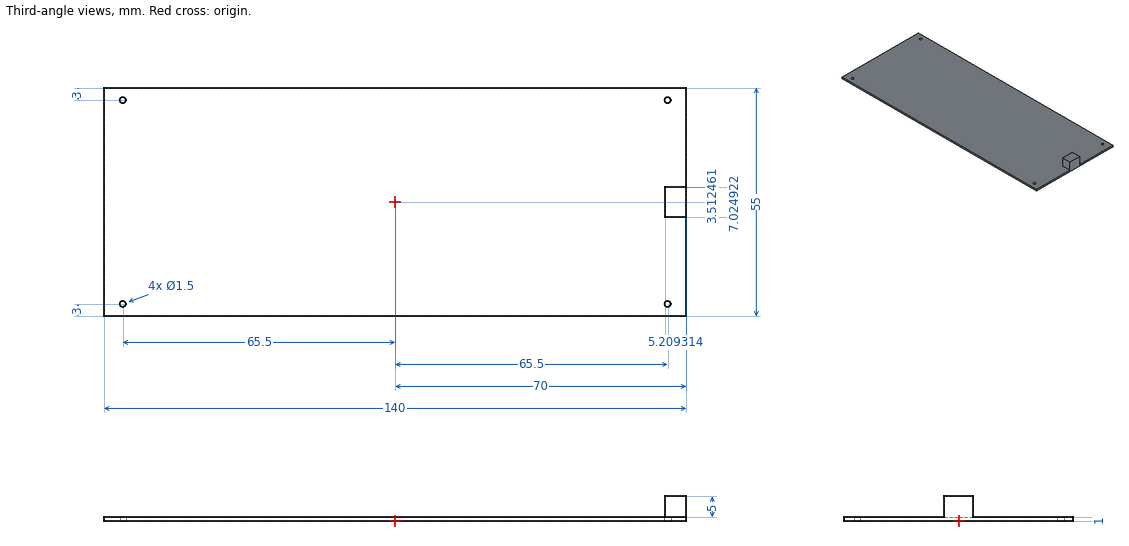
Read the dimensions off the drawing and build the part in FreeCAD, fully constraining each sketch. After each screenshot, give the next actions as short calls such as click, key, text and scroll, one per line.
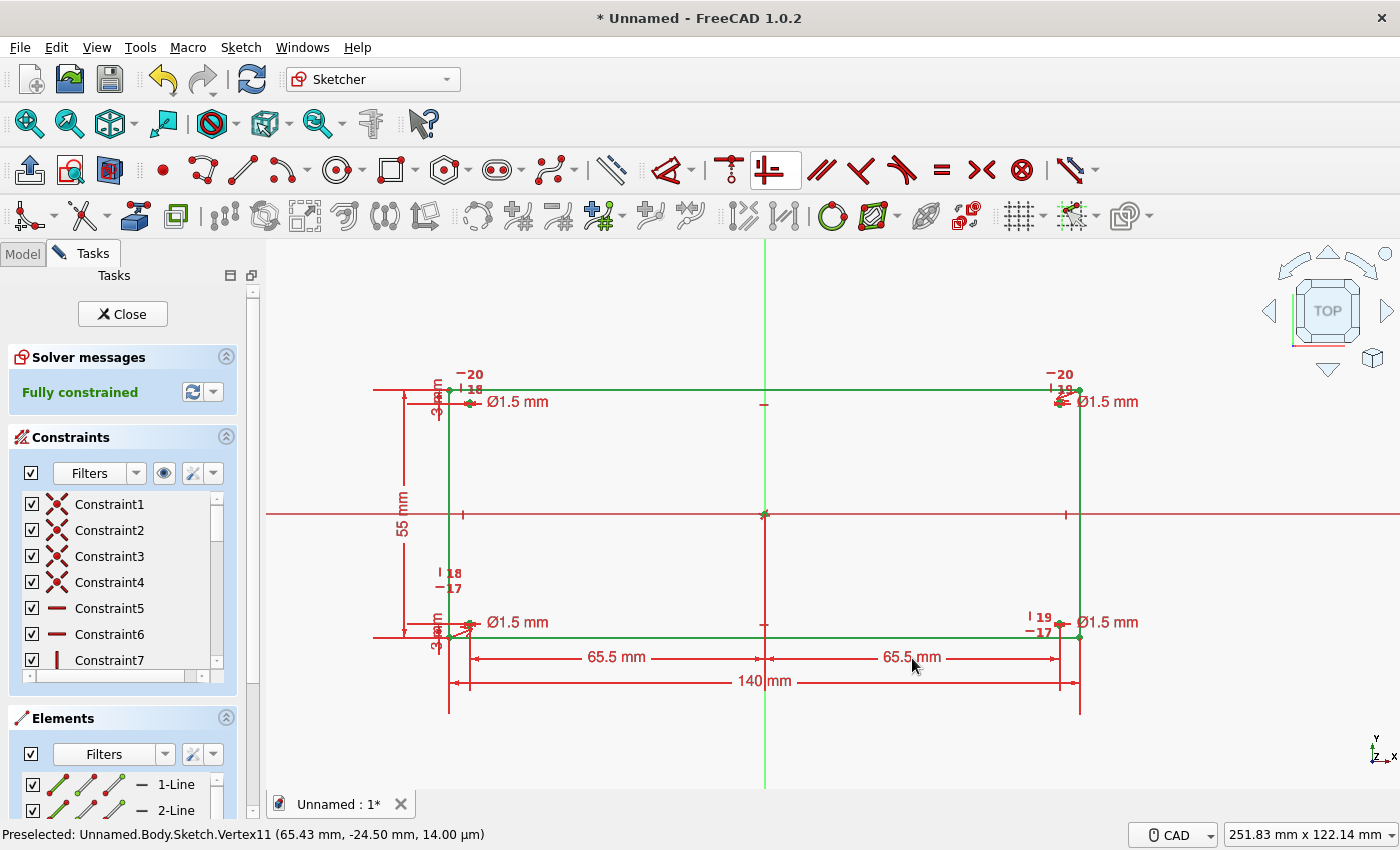
click(123, 314)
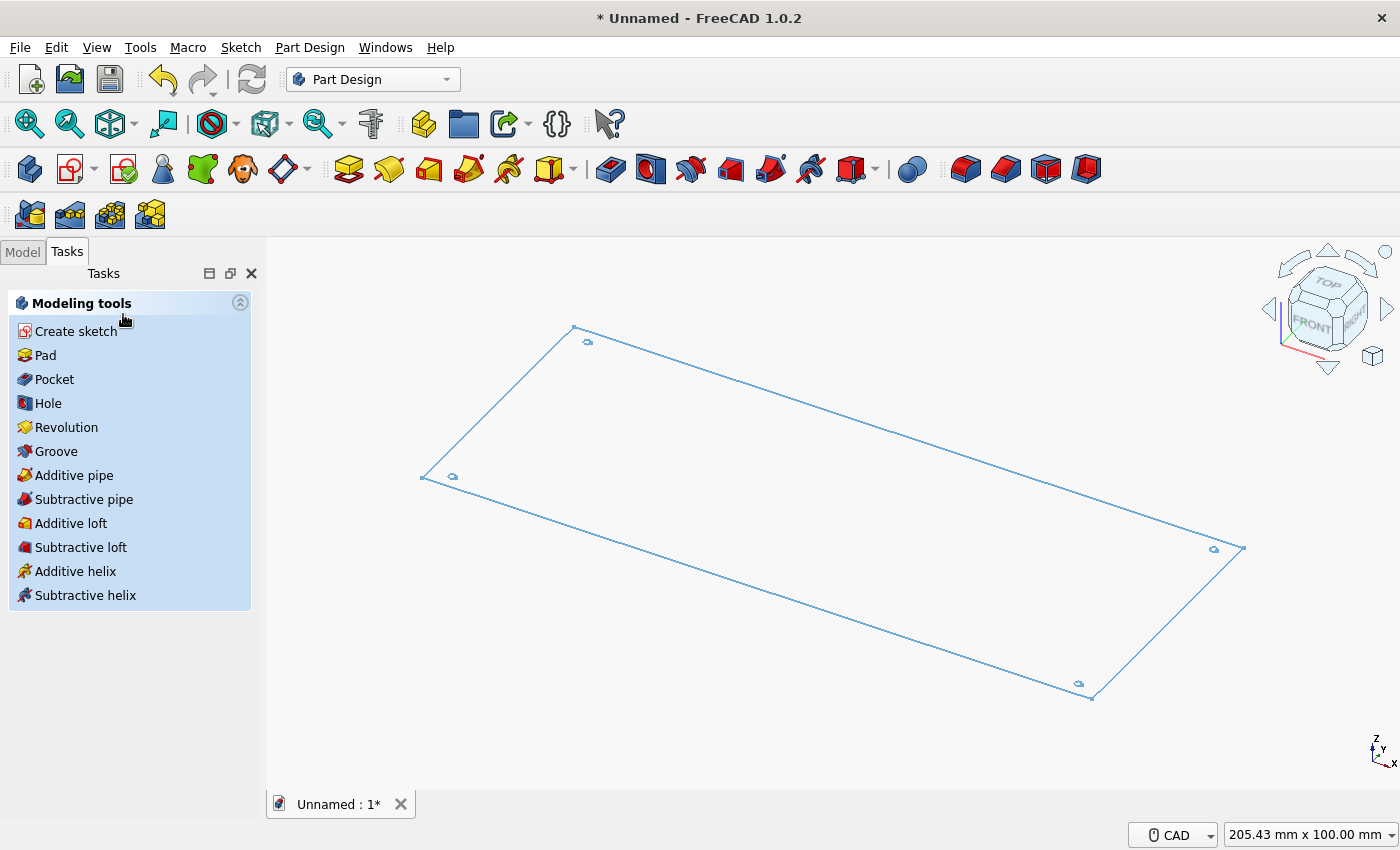
click(350, 170)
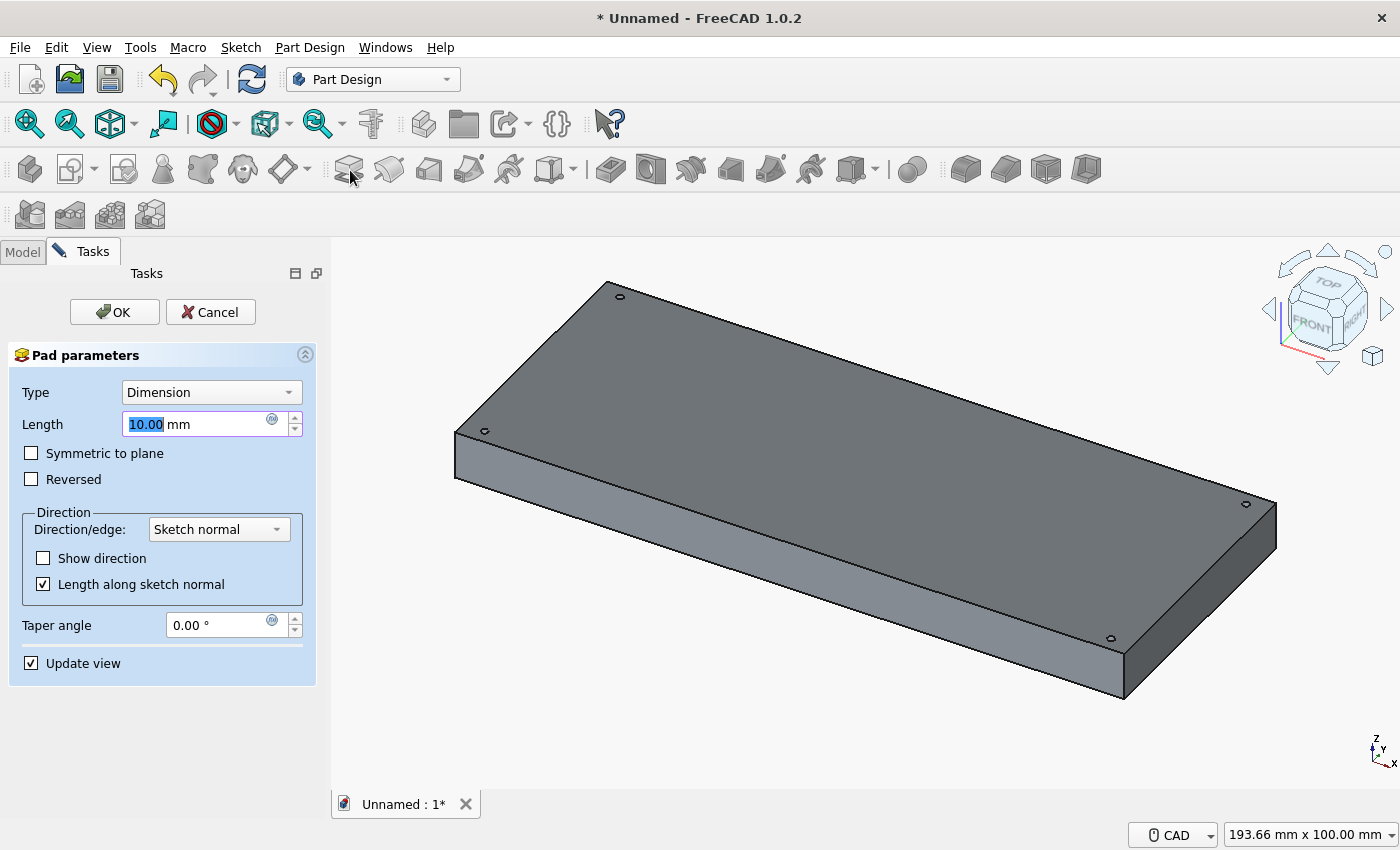
text(1)
key(Tab)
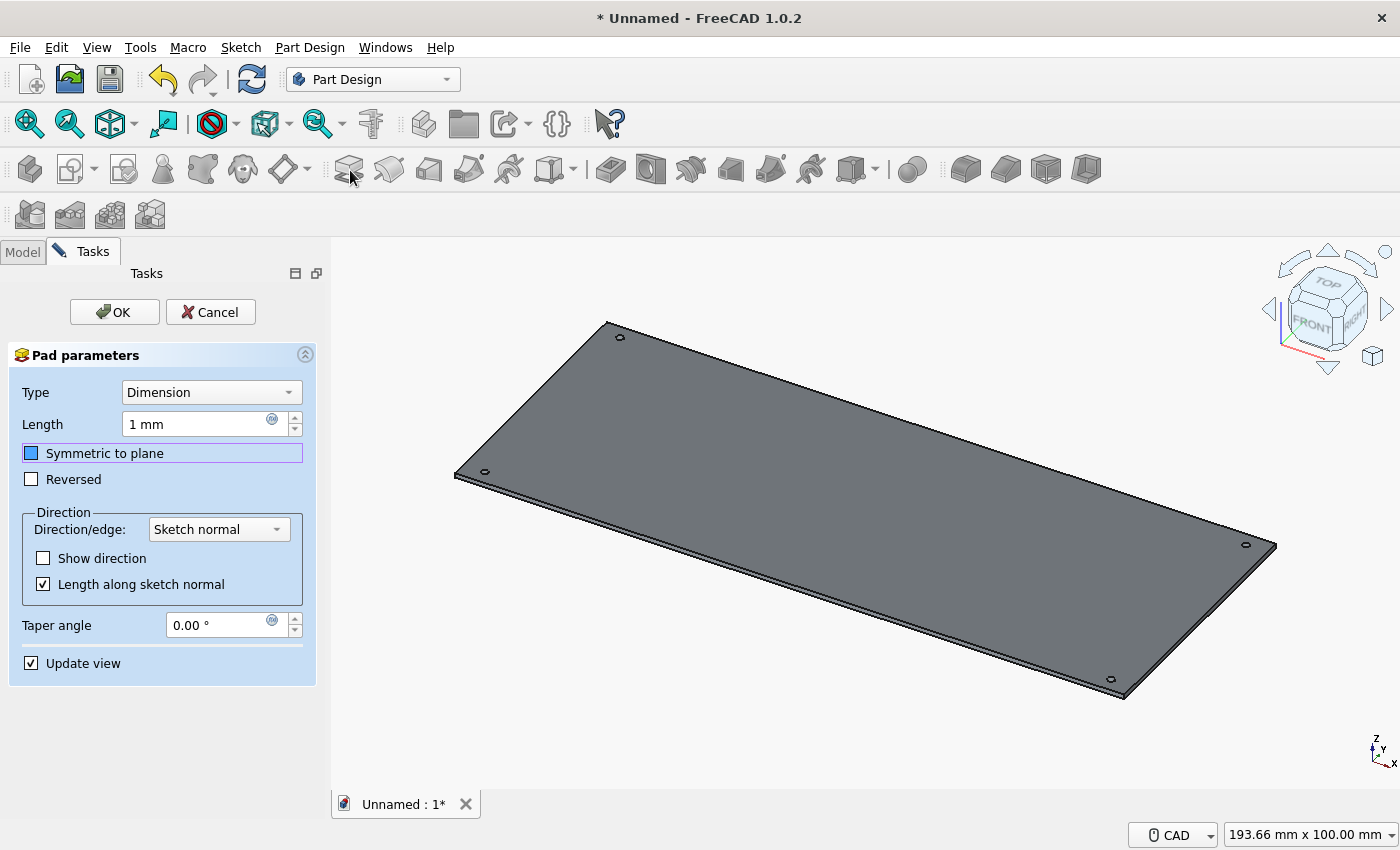
click(115, 312)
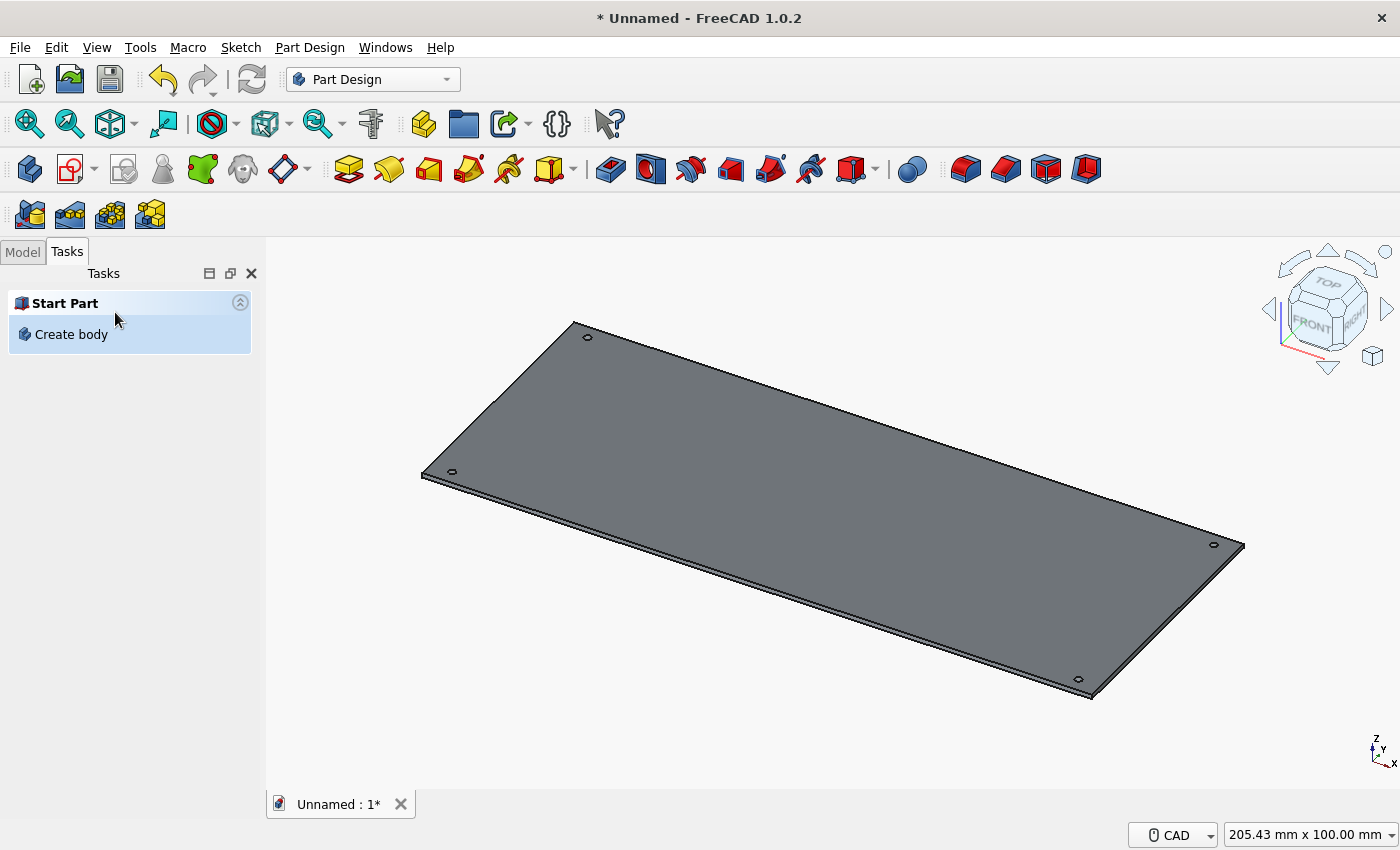
click(1024, 571)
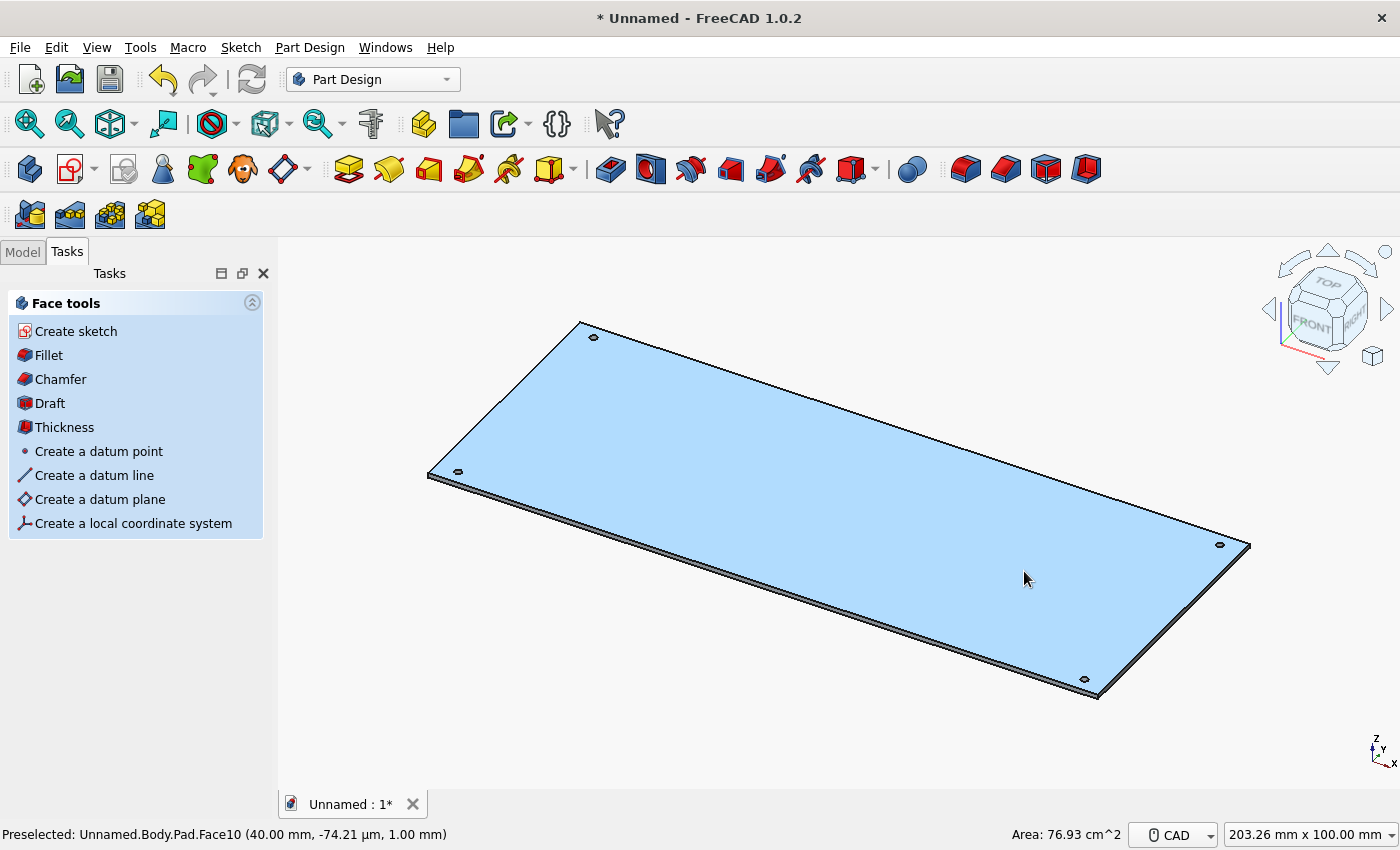
click(70, 170)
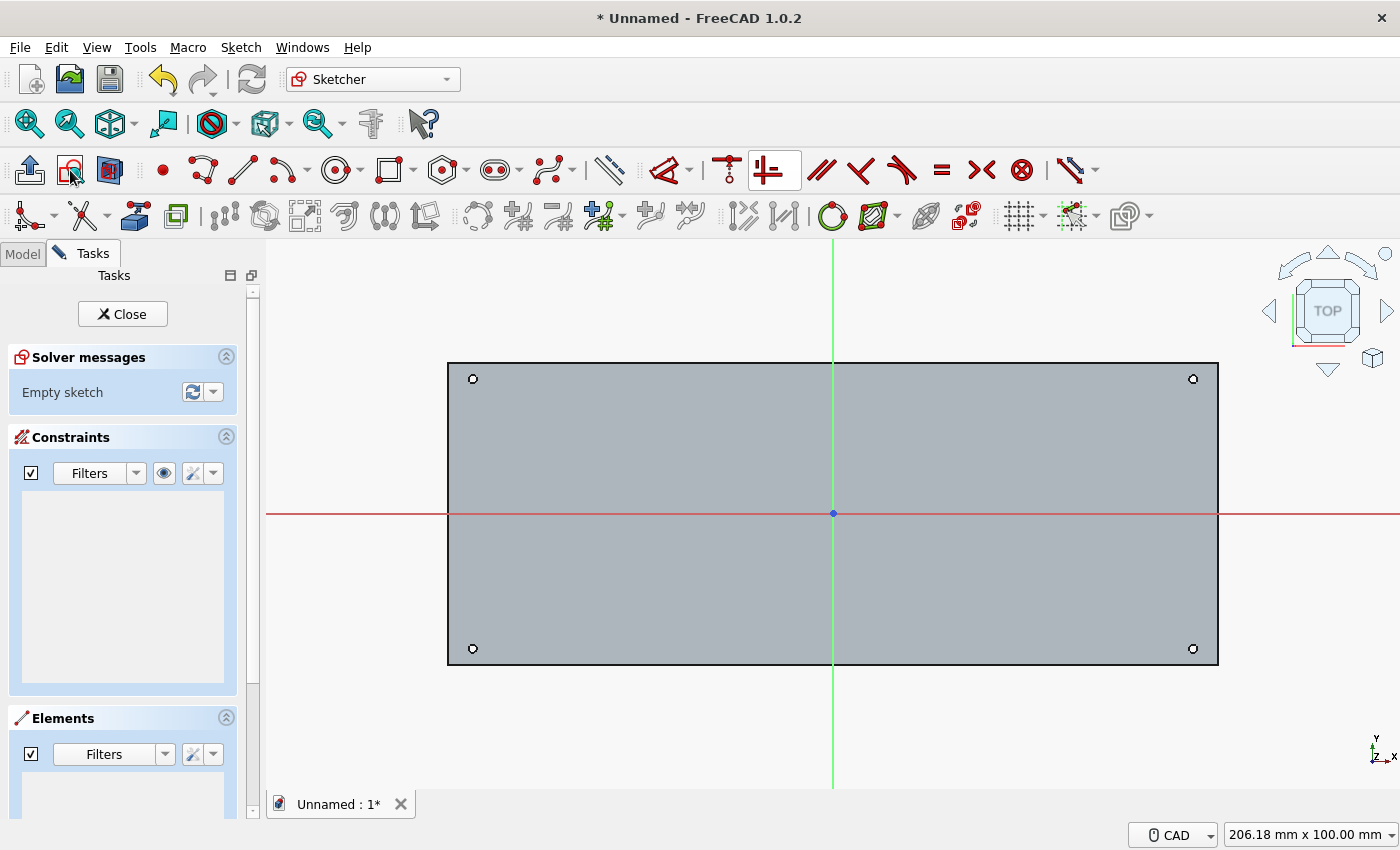
scroll(1235, 514, up, 11)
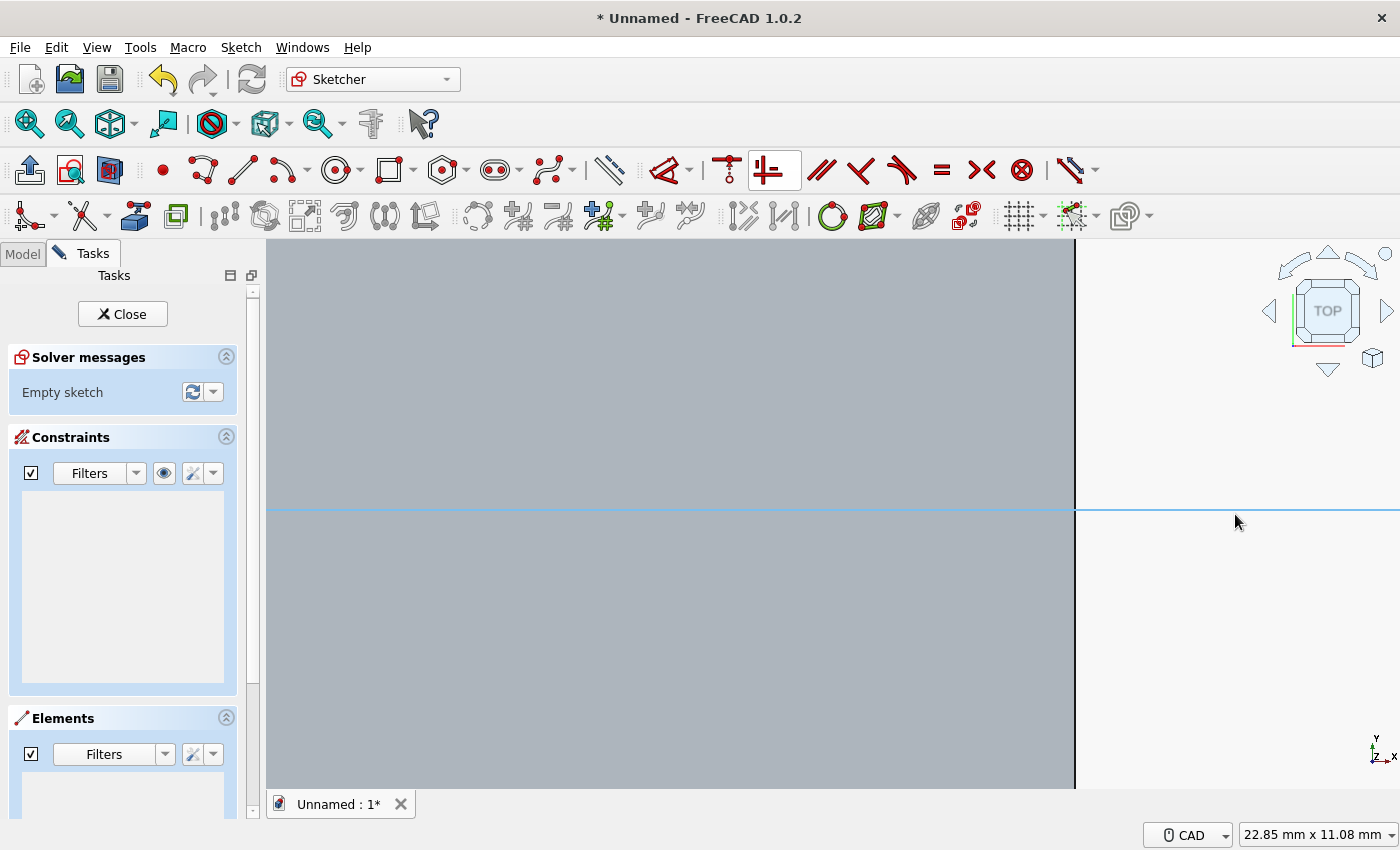
click(390, 170)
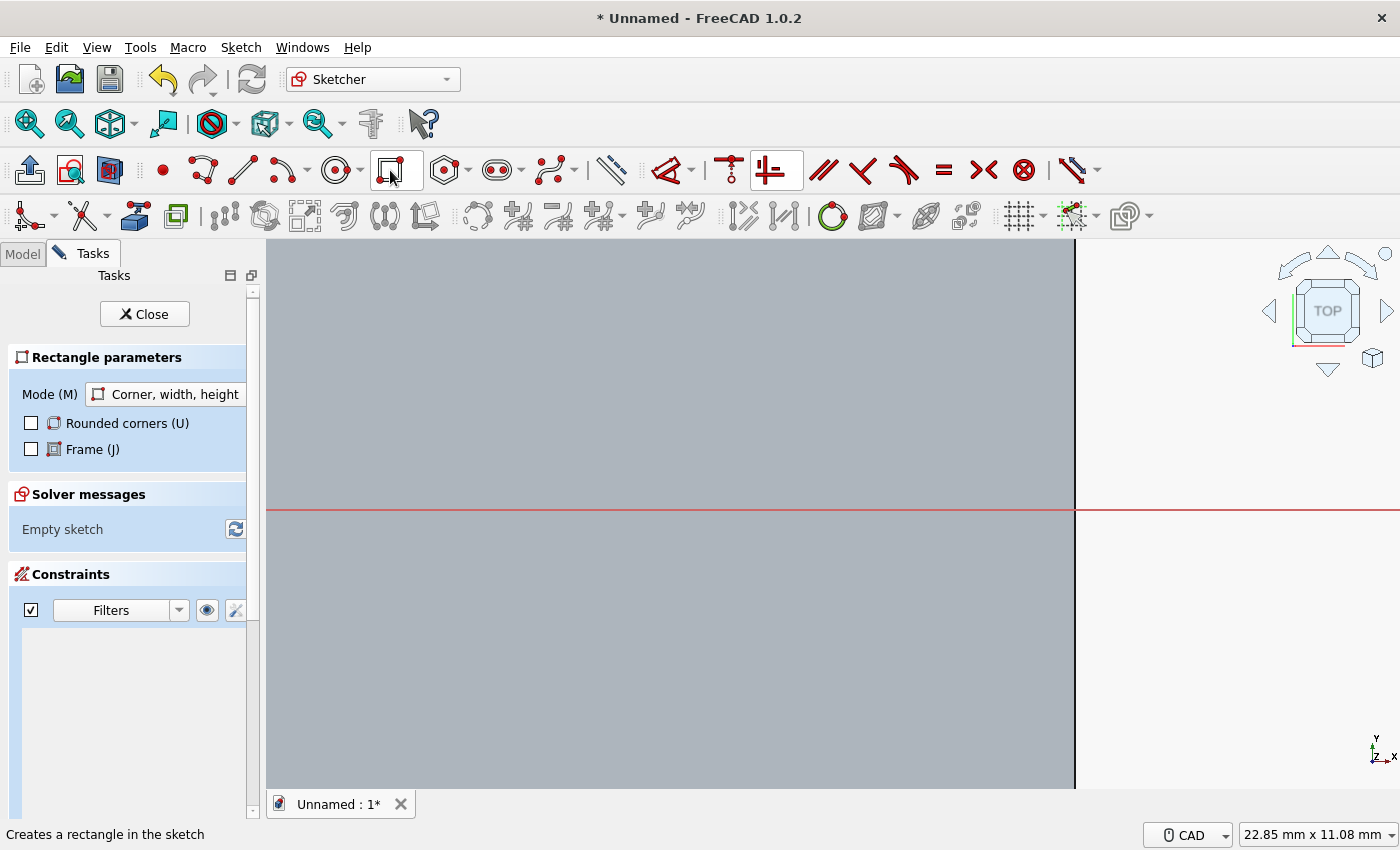
click(816, 336)
move(1075, 684)